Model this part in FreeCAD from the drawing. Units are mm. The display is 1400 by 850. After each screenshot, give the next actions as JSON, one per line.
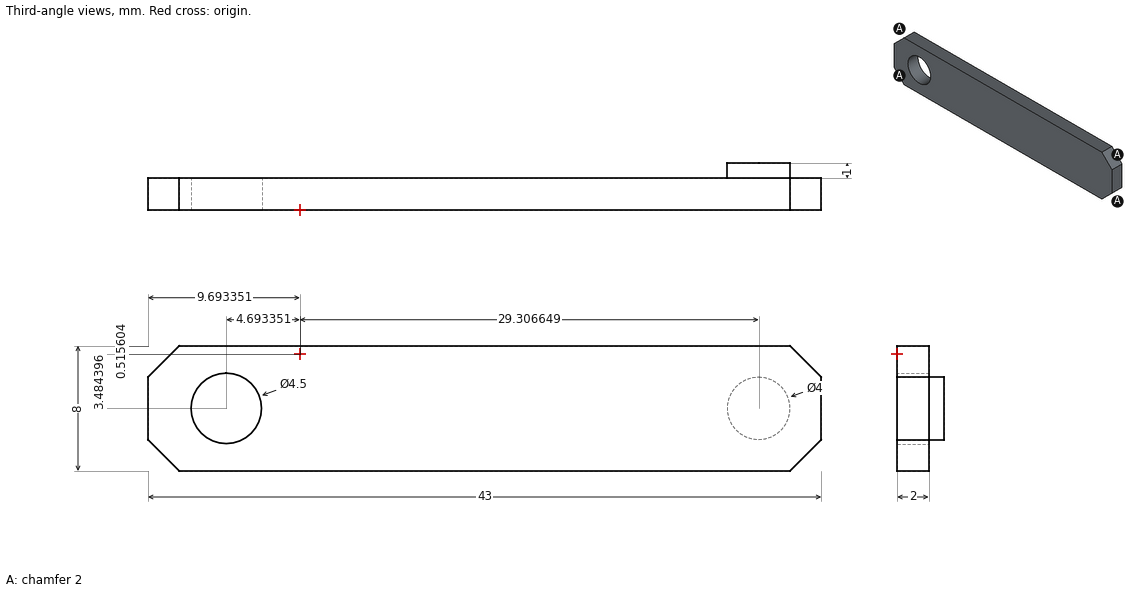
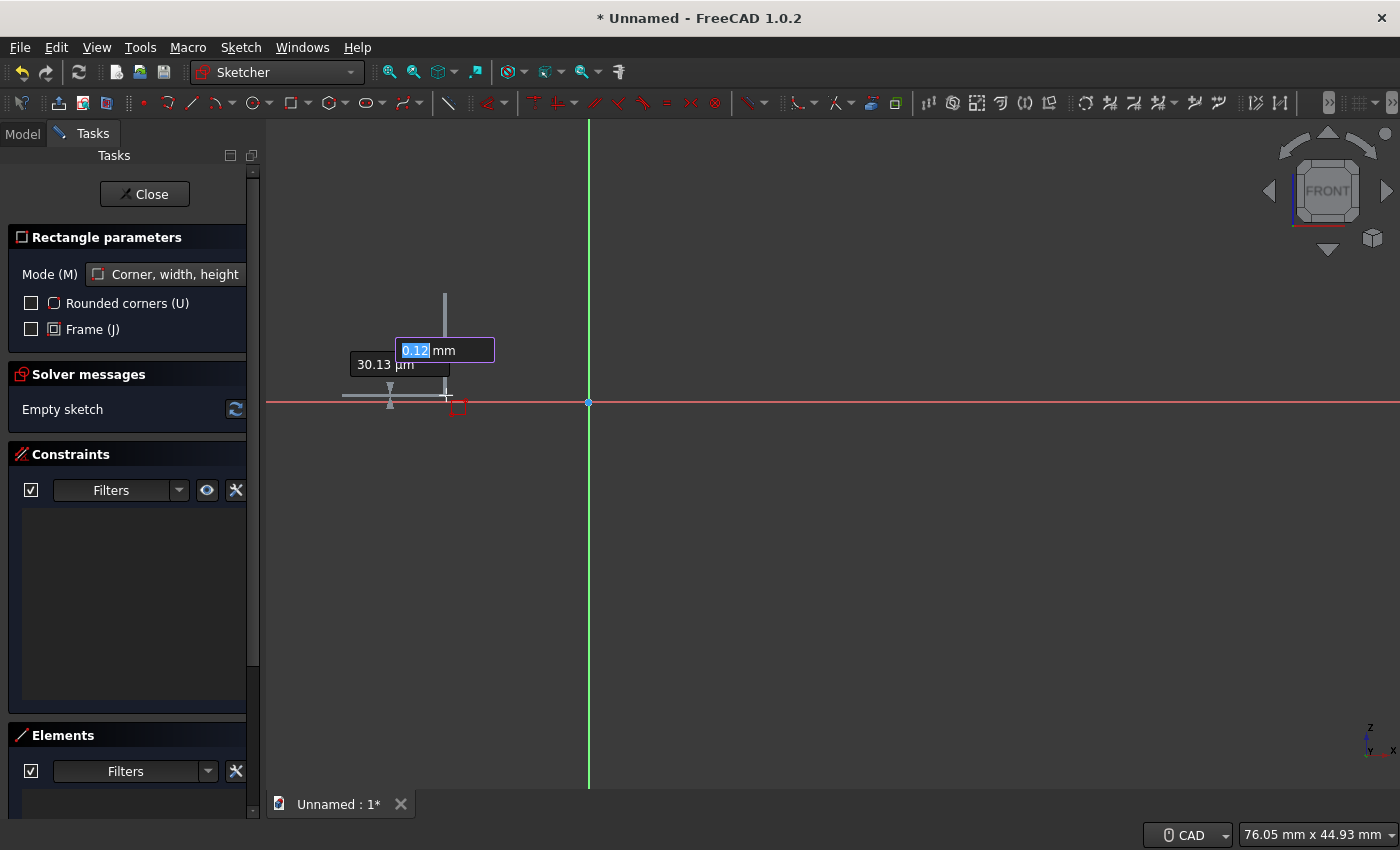
{"action": "left_click", "coordinate": [1085, 514]}
{"action": "key", "text": "Escape"}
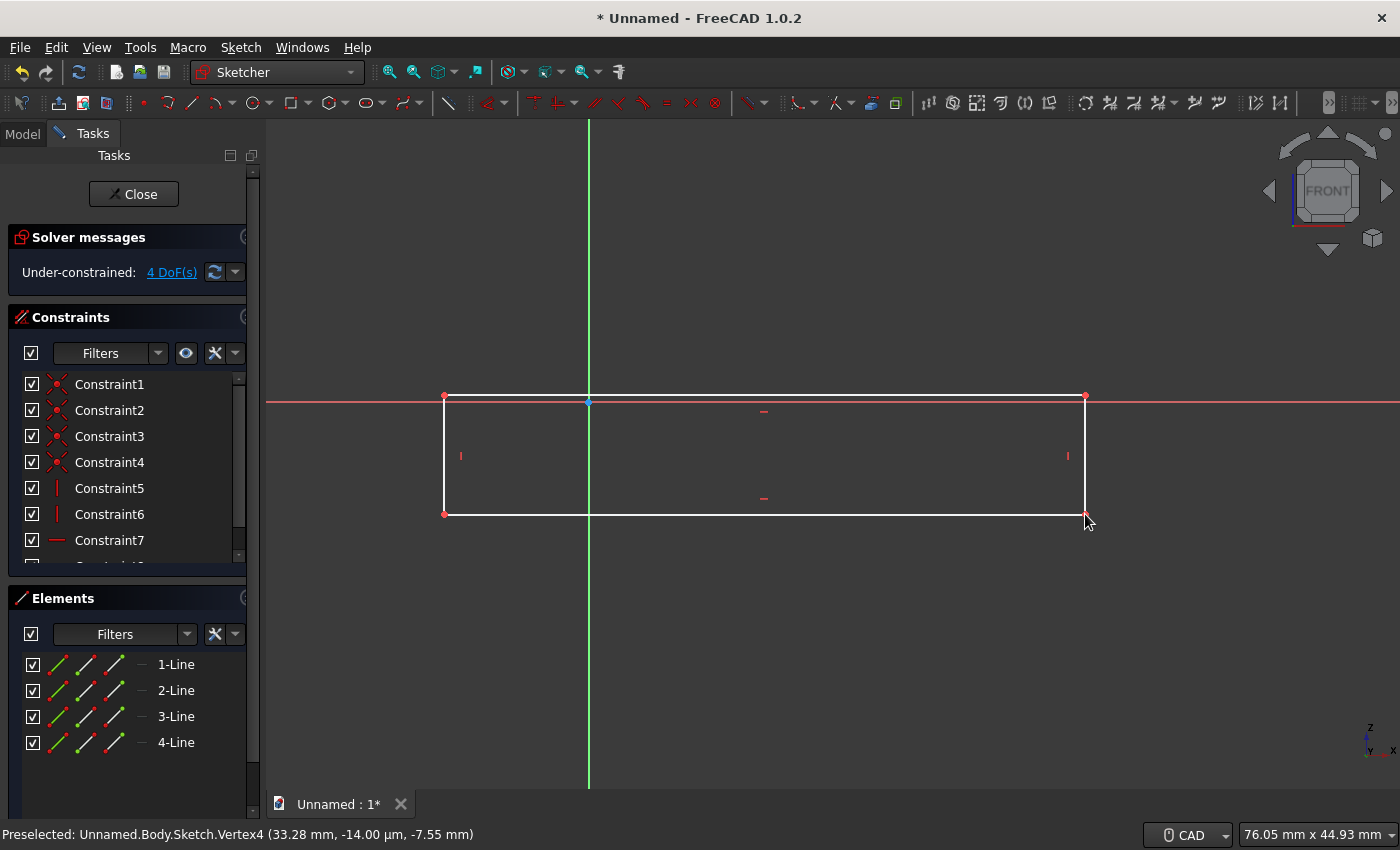
{"action": "left_click", "coordinate": [488, 104]}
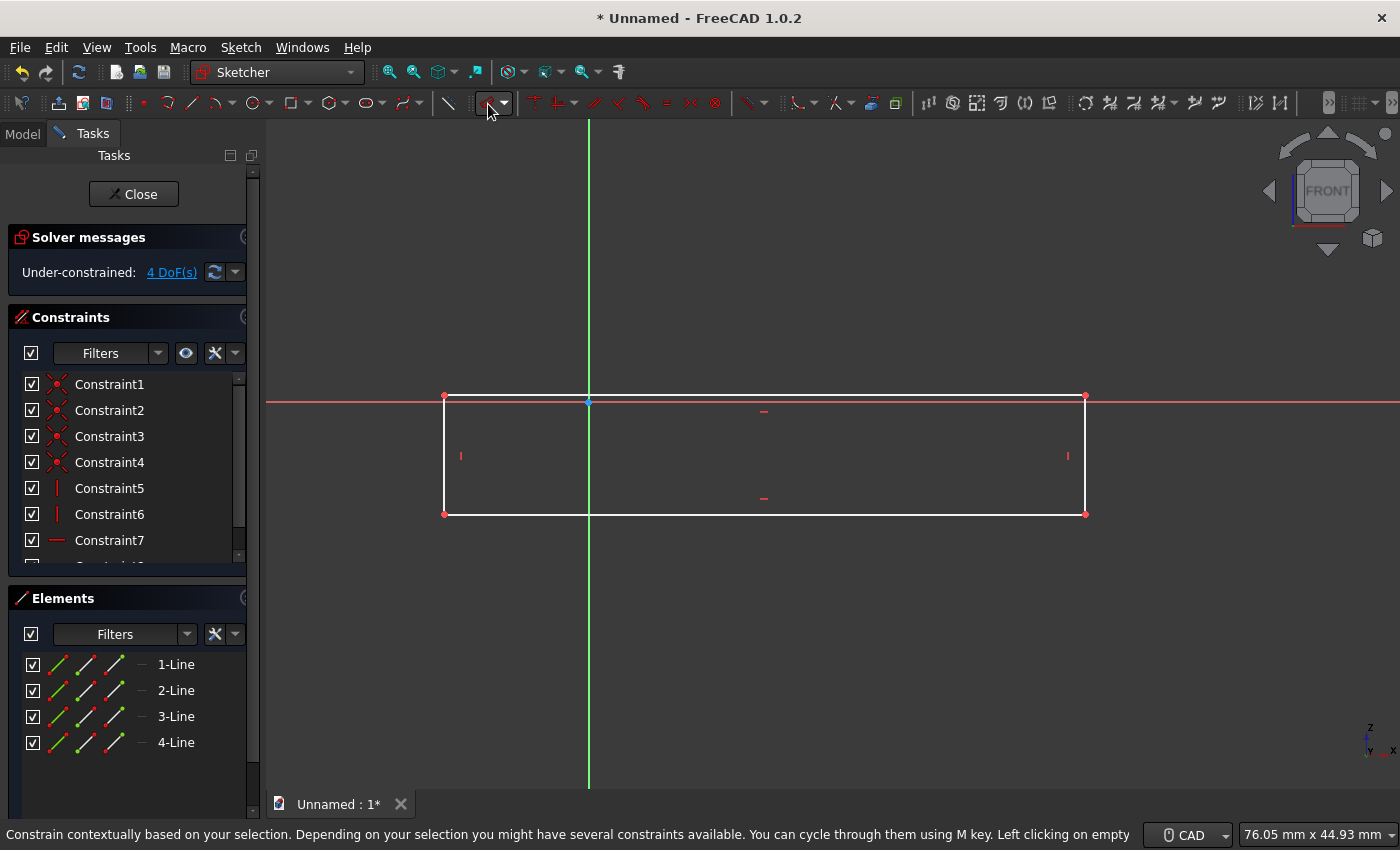
{"action": "left_click", "coordinate": [444, 431]}
{"action": "left_click", "coordinate": [410, 455]}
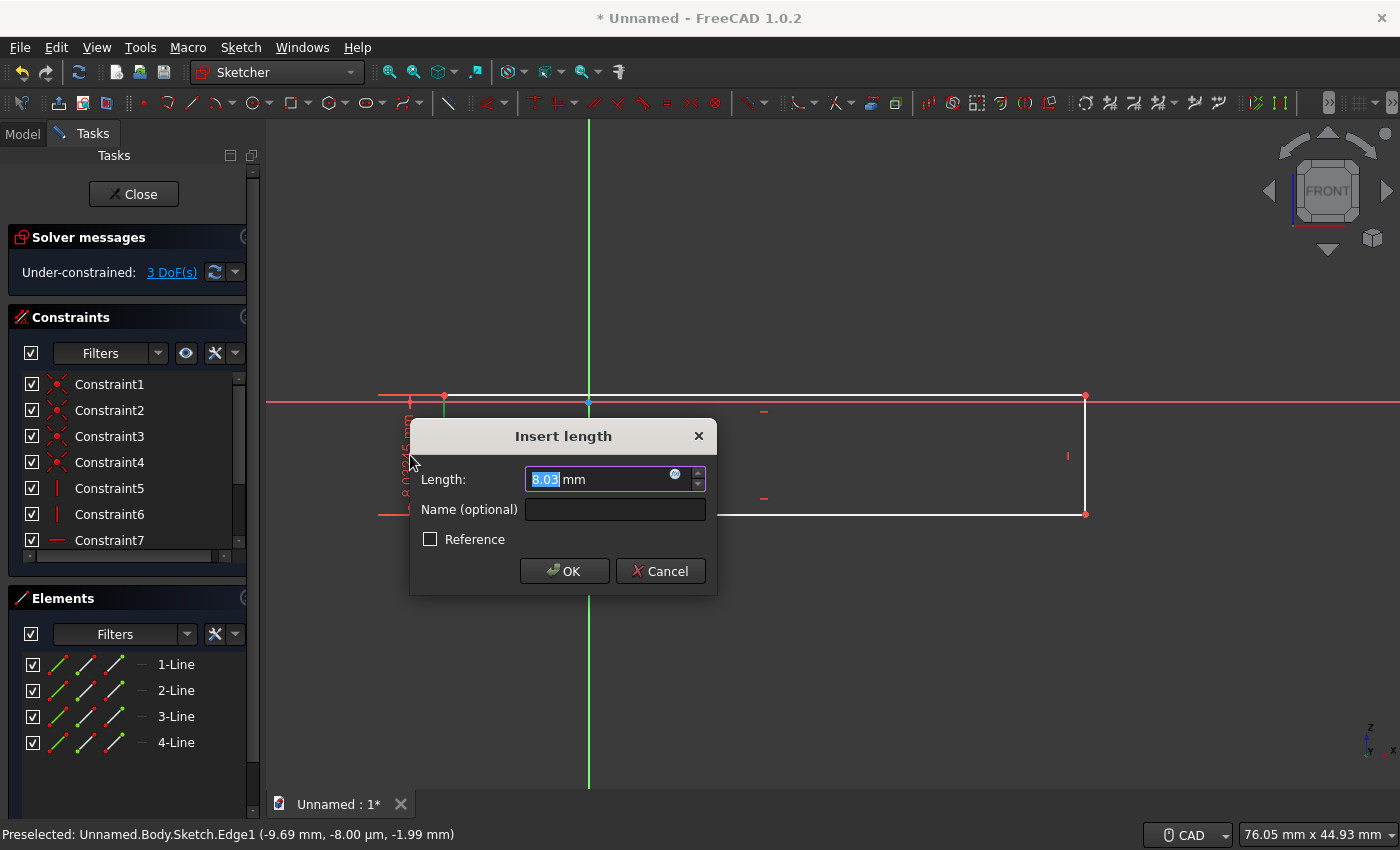
{"action": "type", "text": "8"}
{"action": "key", "text": "Return"}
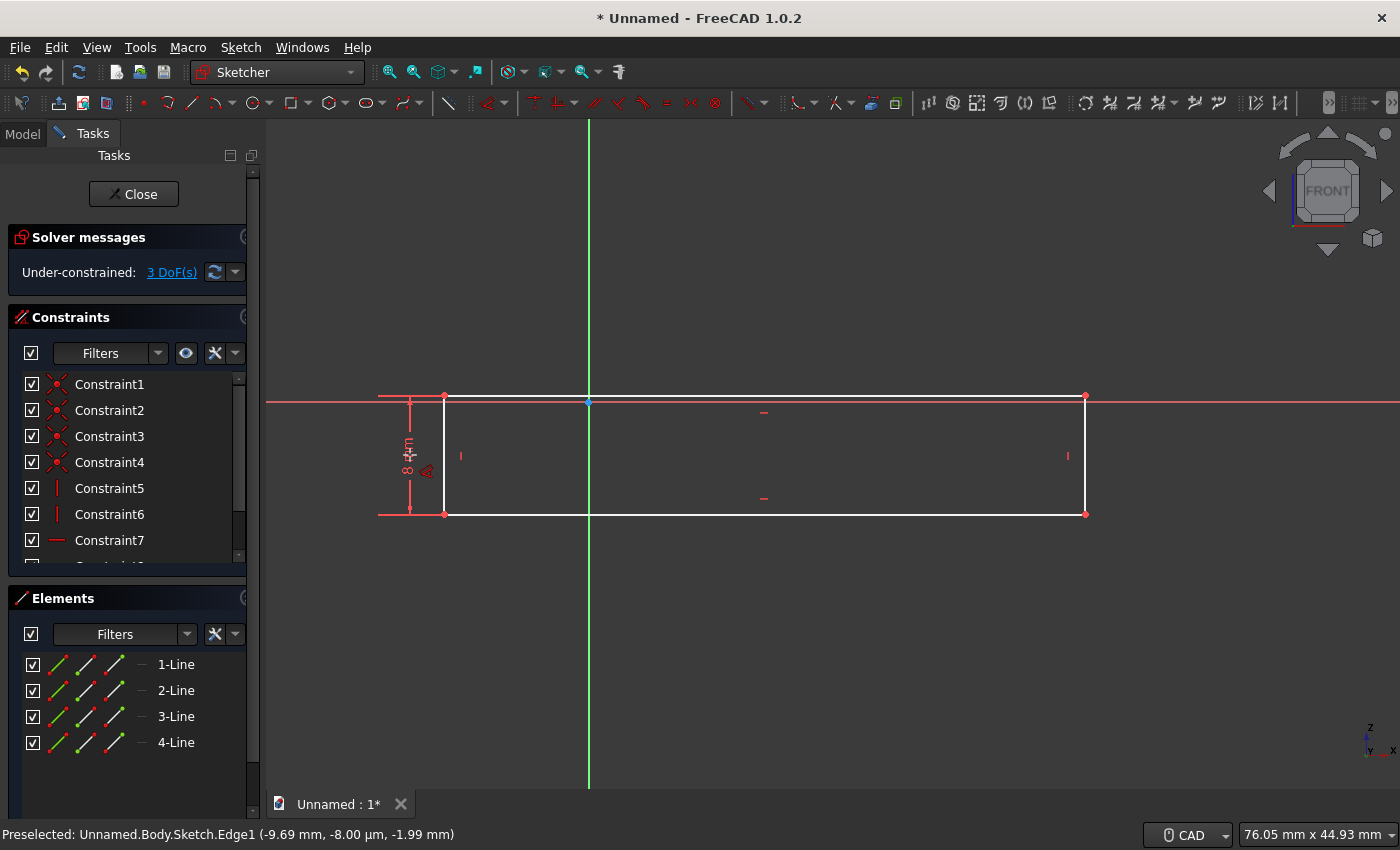
{"action": "left_click", "coordinate": [637, 515]}
{"action": "left_click", "coordinate": [765, 549]}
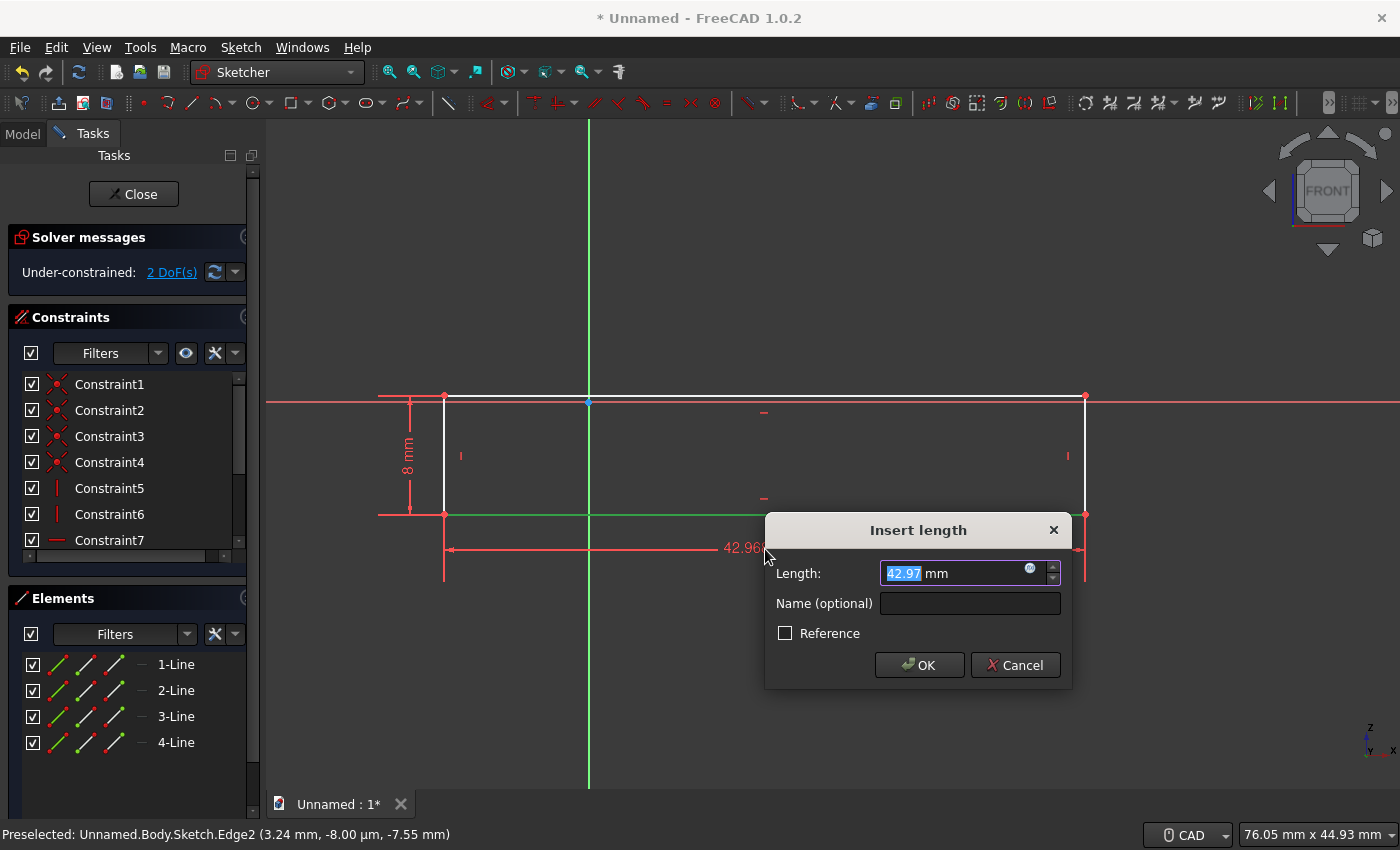
{"action": "type", "text": "43"}
{"action": "key", "text": "Return"}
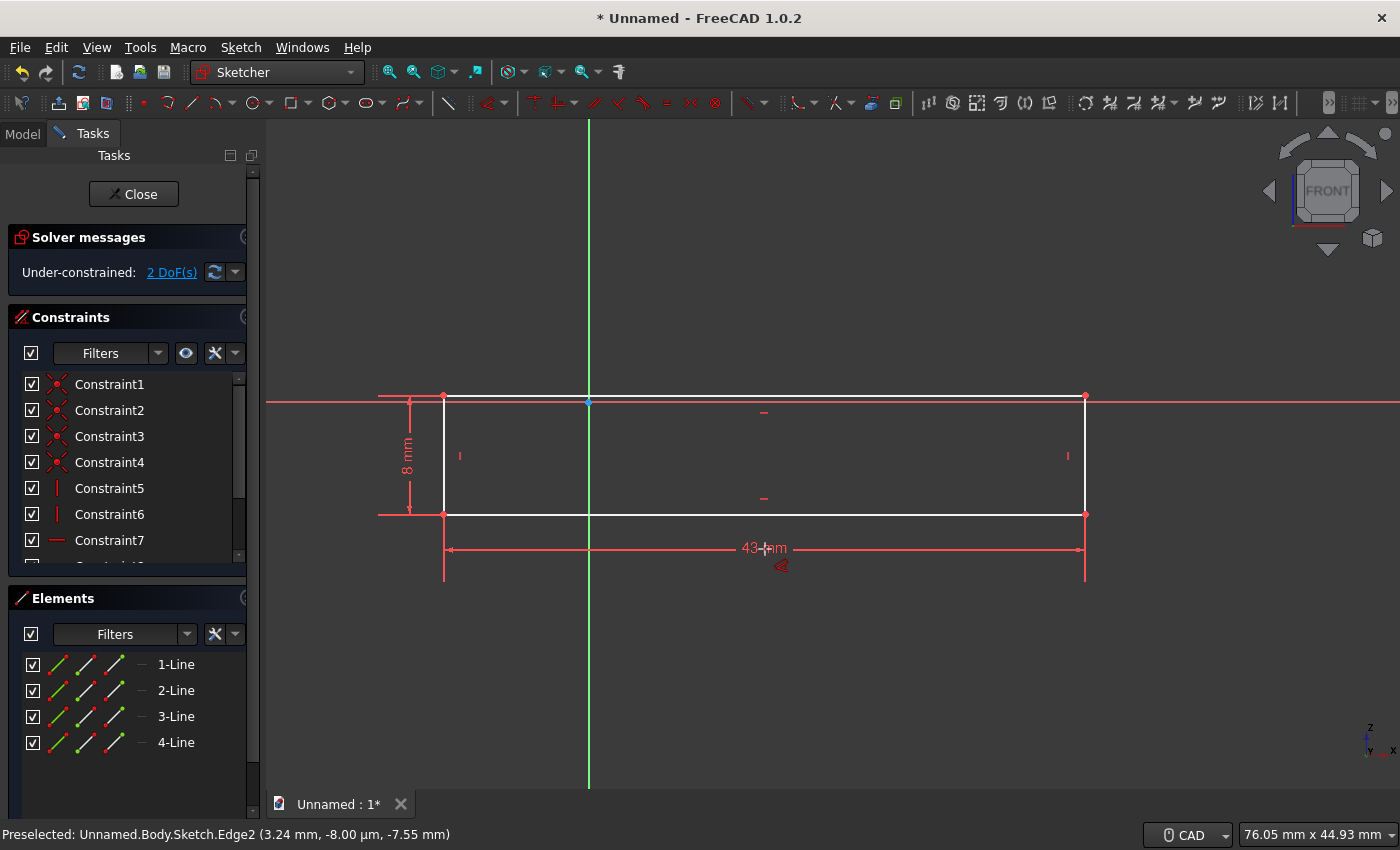
{"action": "left_click", "coordinate": [444, 396]}
{"action": "left_click", "coordinate": [516, 362]}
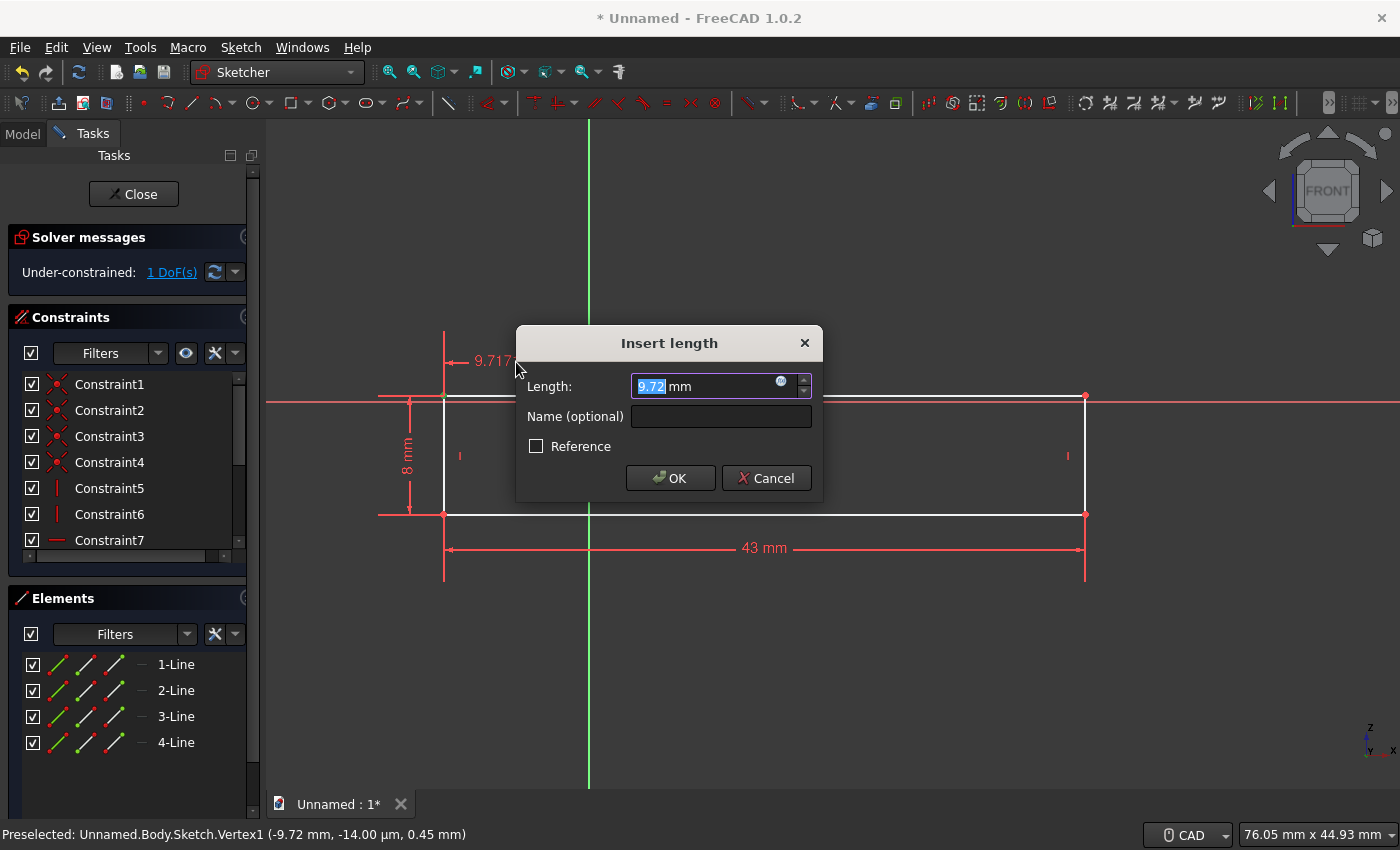
{"action": "type", "text": "9.693351"}
{"action": "key", "text": "Return"}